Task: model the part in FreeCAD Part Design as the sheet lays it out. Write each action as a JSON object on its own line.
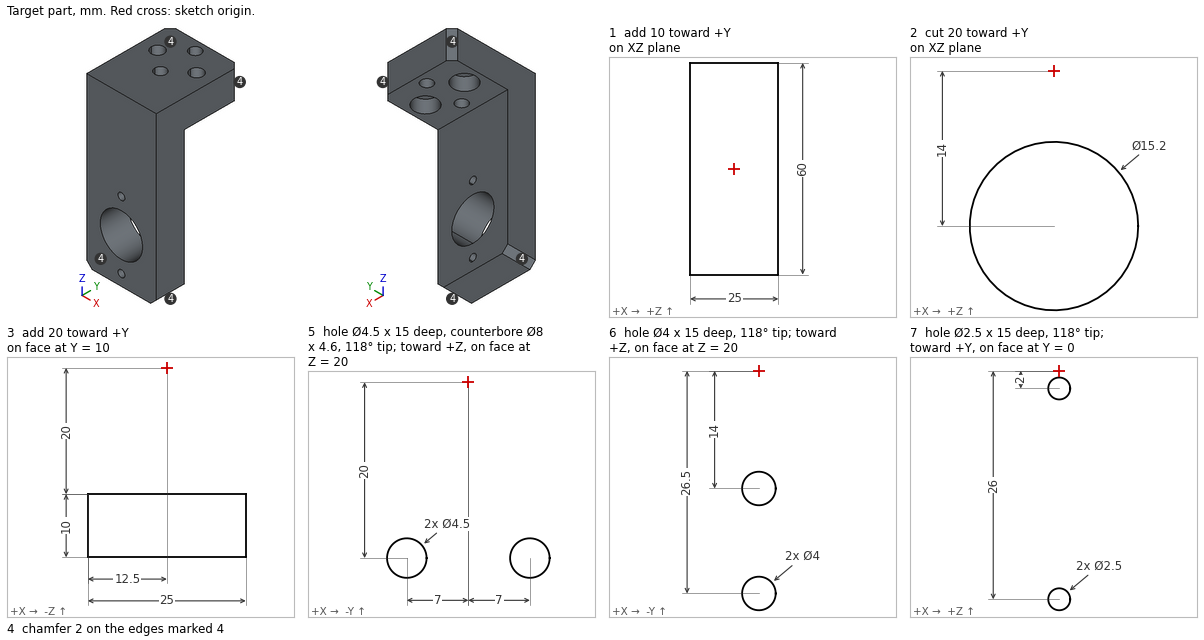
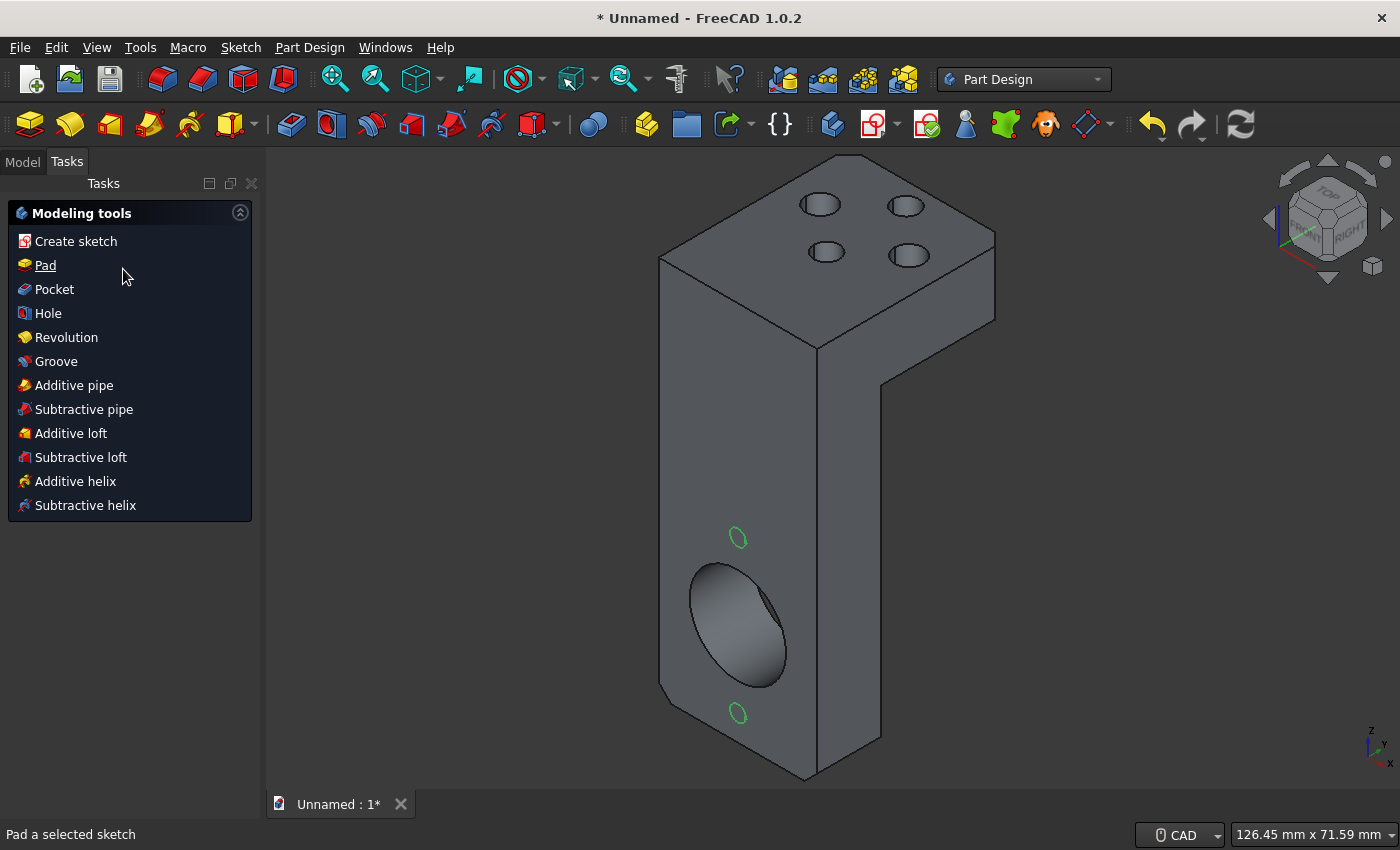
{"action": "left_click", "coordinate": [332, 124]}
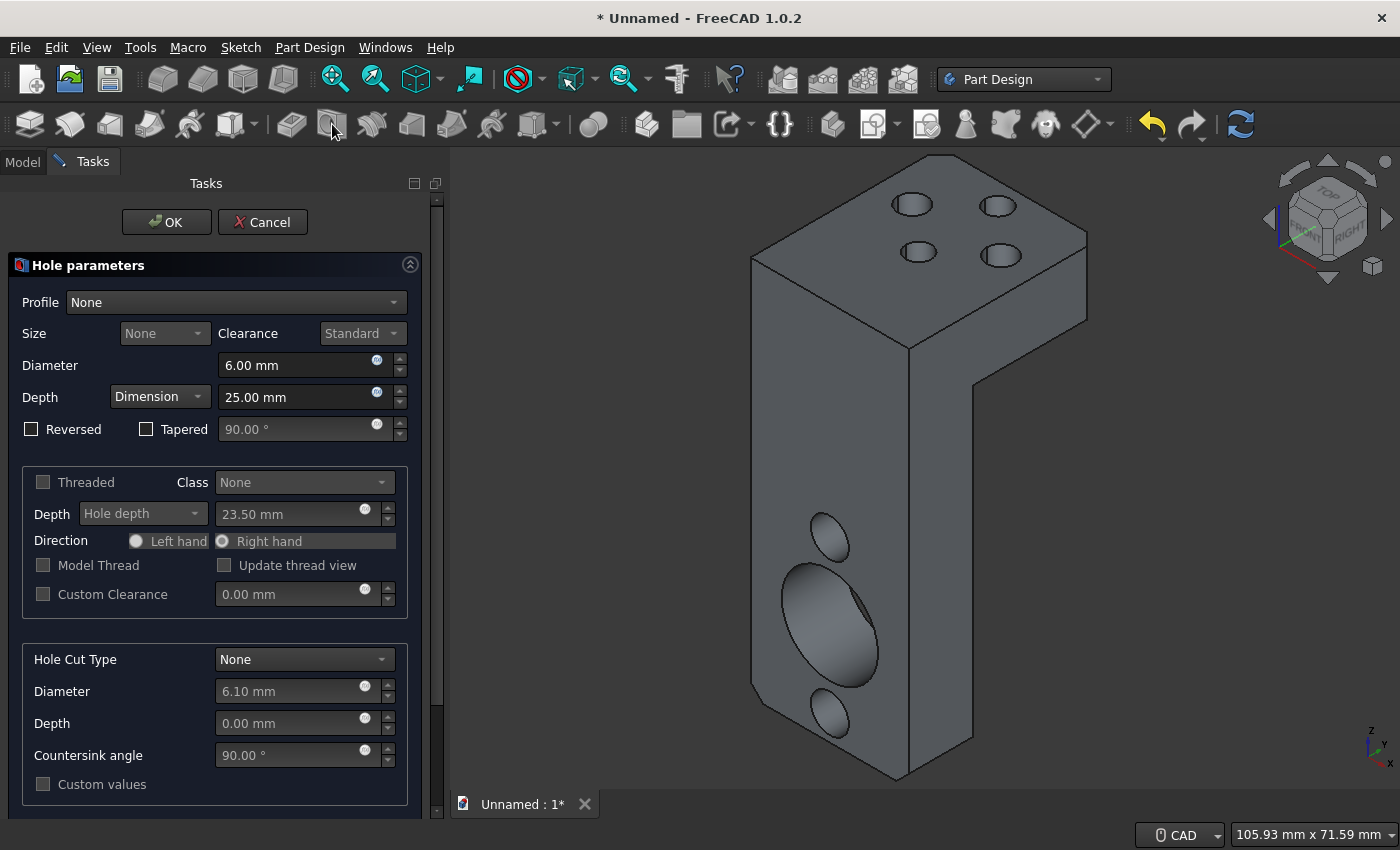
{"action": "triple_click", "coordinate": [305, 365]}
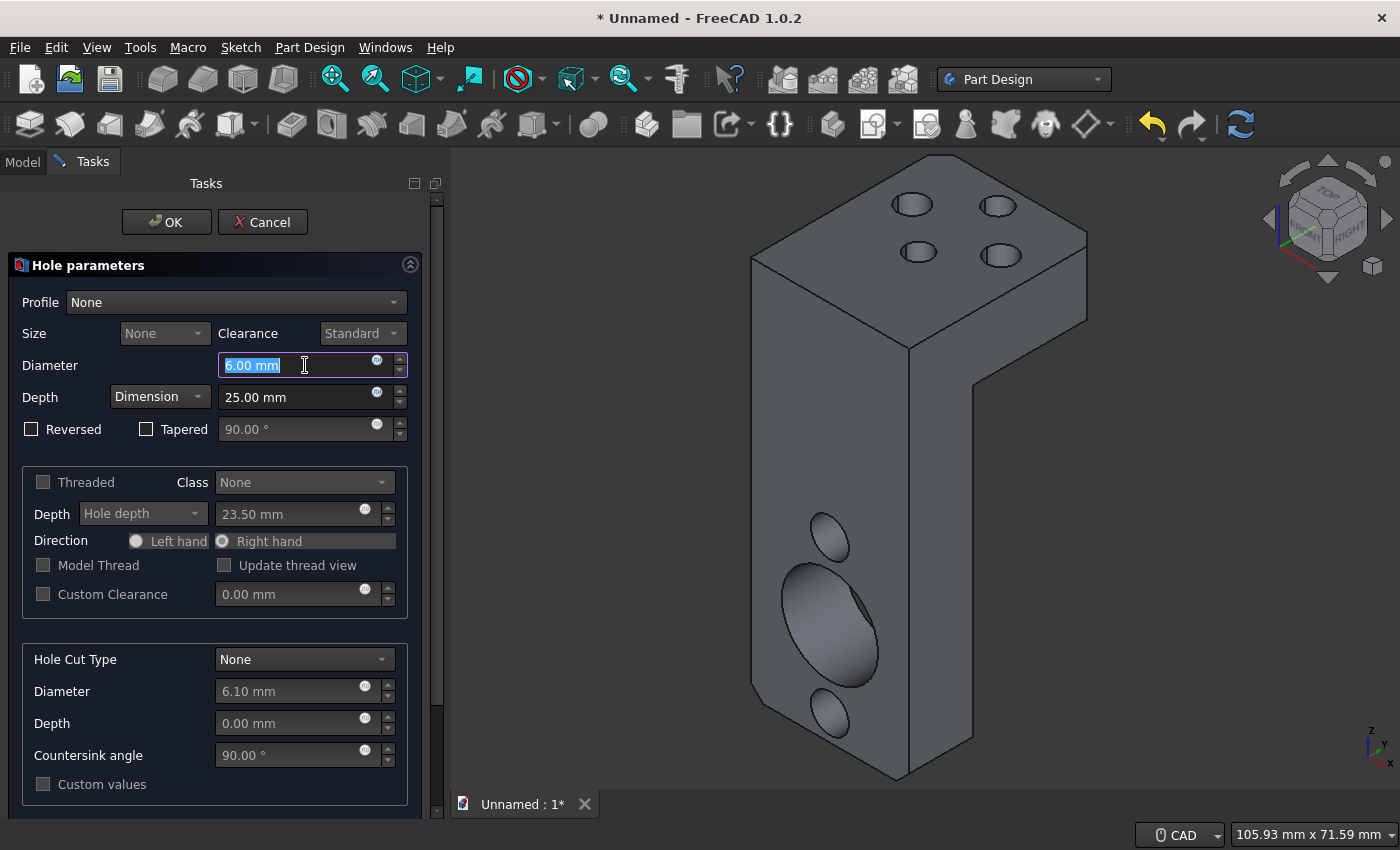
{"action": "type", "text": "2.5"}
{"action": "key", "text": "Tab"}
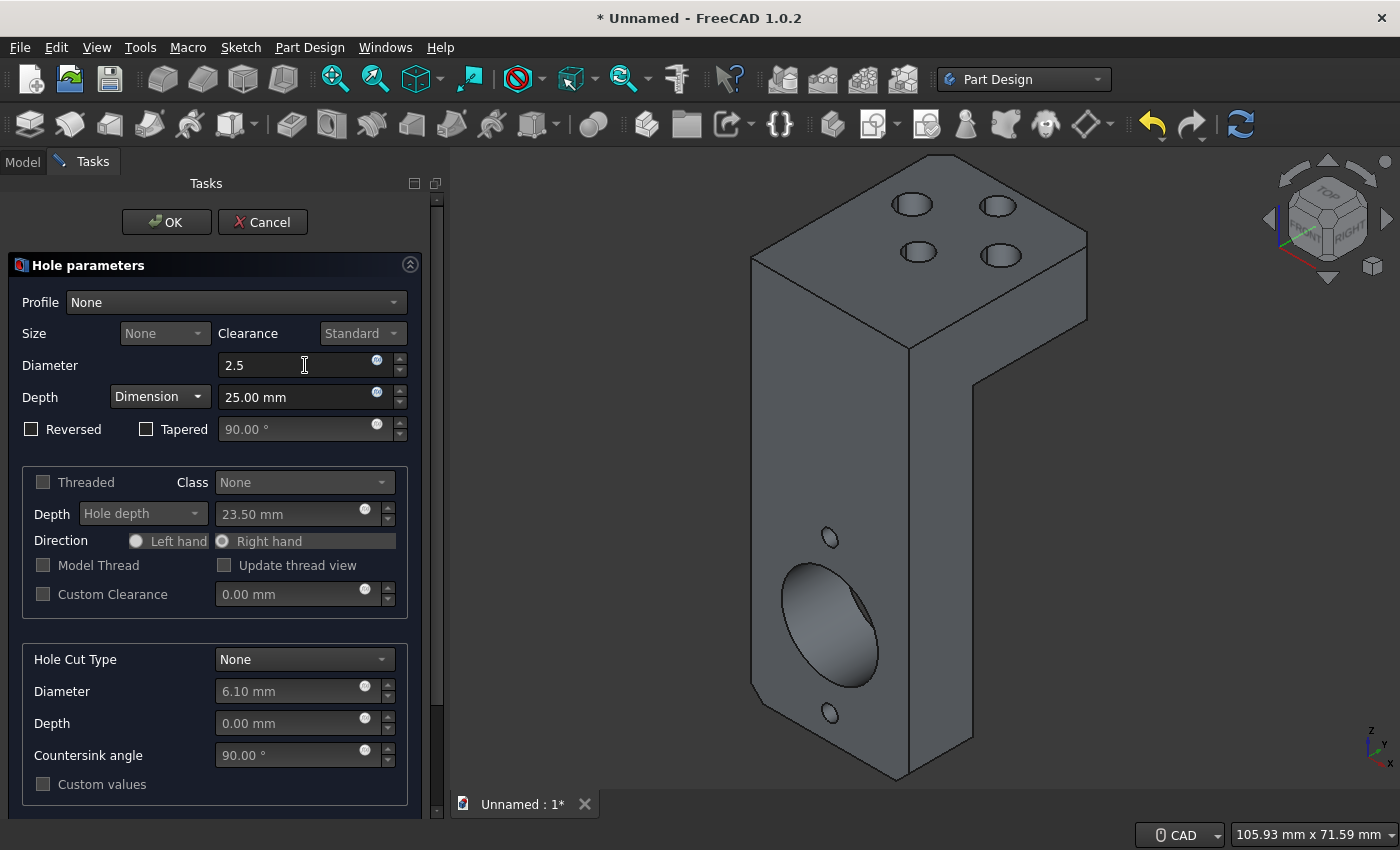
{"action": "triple_click", "coordinate": [305, 397]}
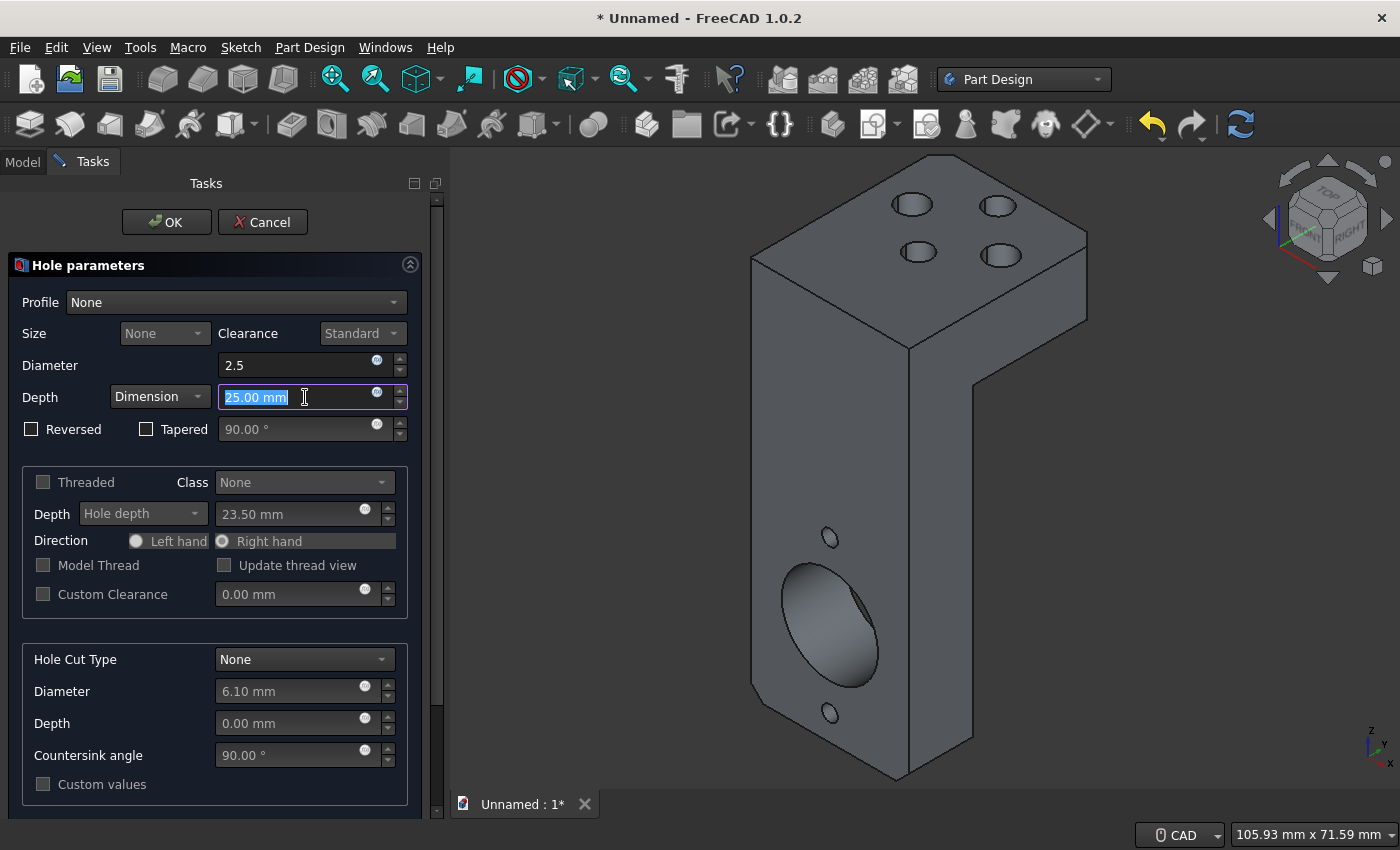
{"action": "type", "text": "15"}
{"action": "key", "text": "Tab"}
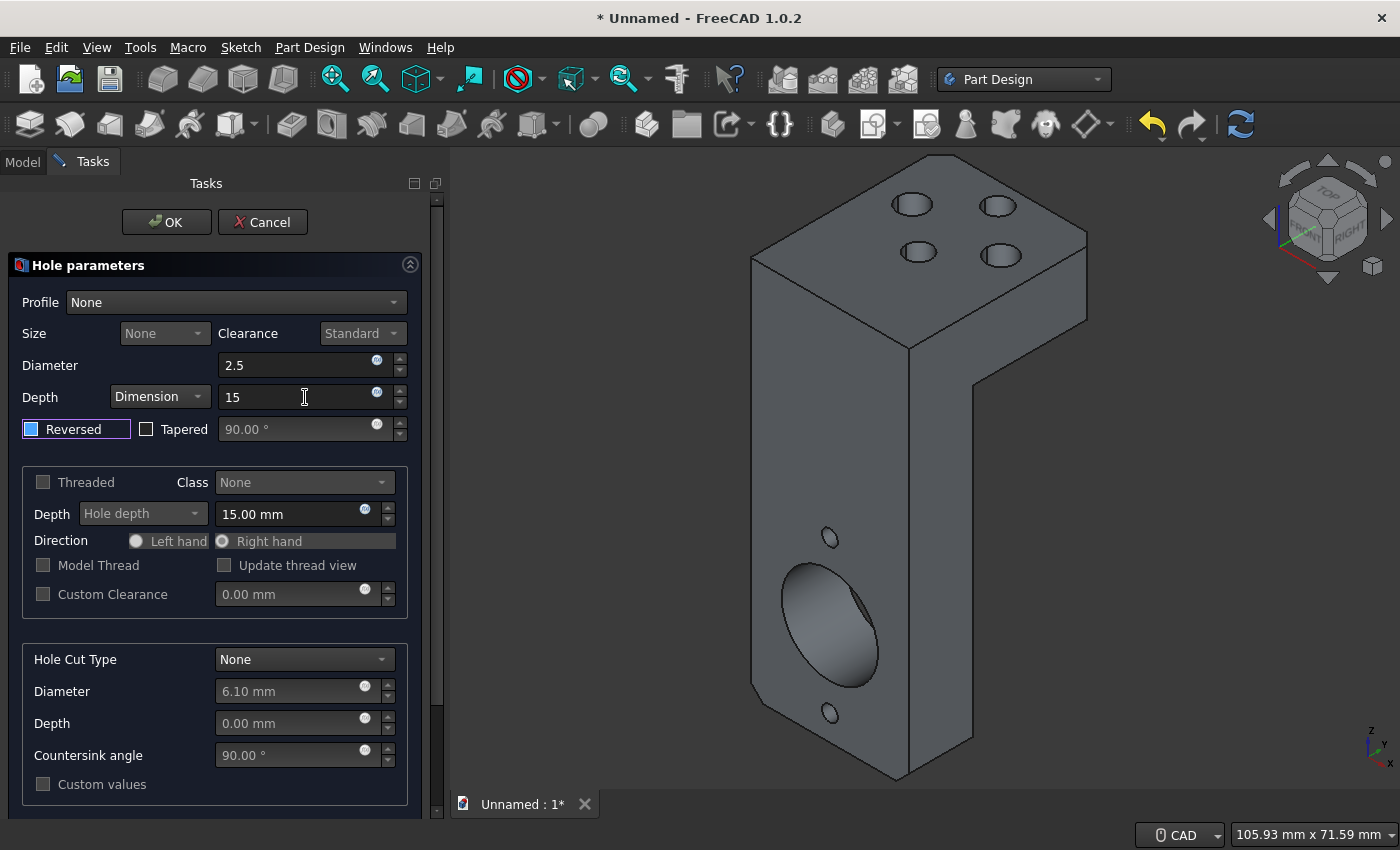
{"action": "left_click", "coordinate": [167, 222]}